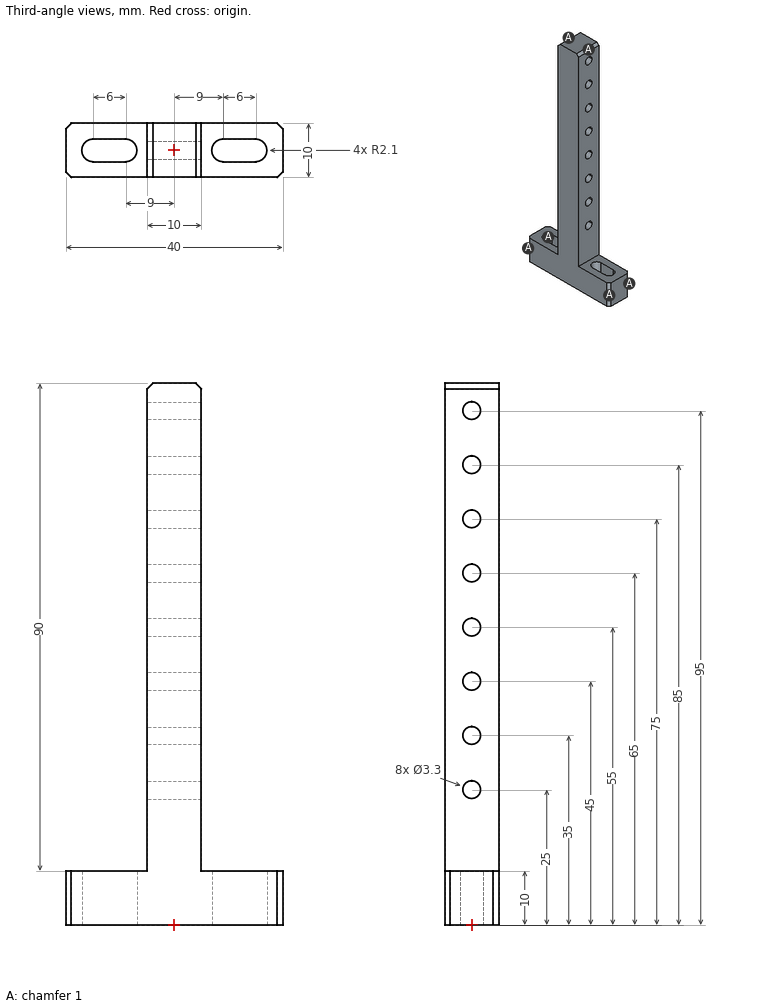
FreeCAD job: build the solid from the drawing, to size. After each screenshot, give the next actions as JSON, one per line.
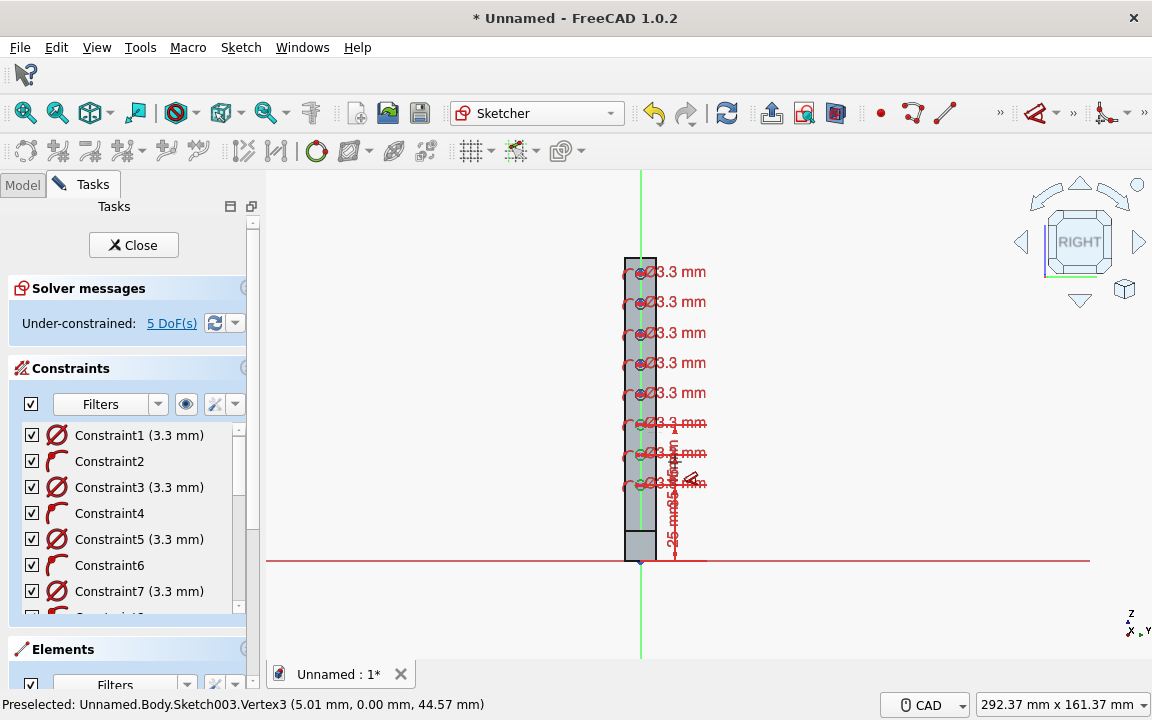
{"action": "left_click", "coordinate": [641, 395]}
{"action": "left_click", "coordinate": [675, 440]}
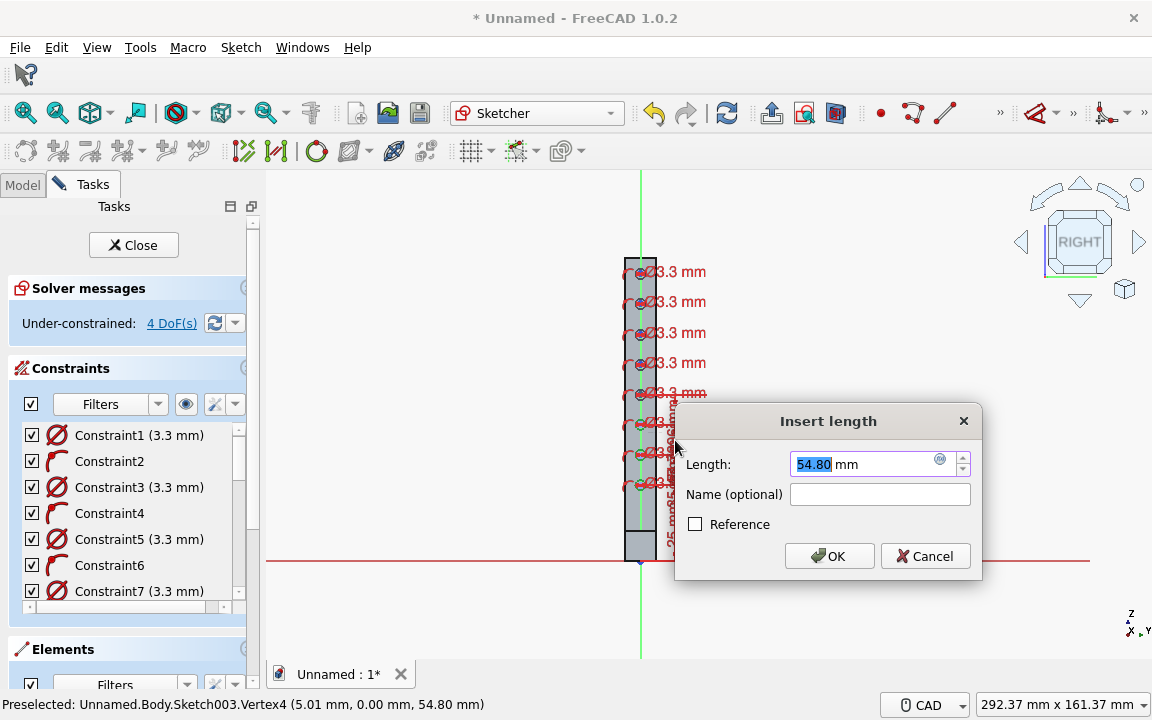
{"action": "type", "text": "55"}
{"action": "key", "text": "Return"}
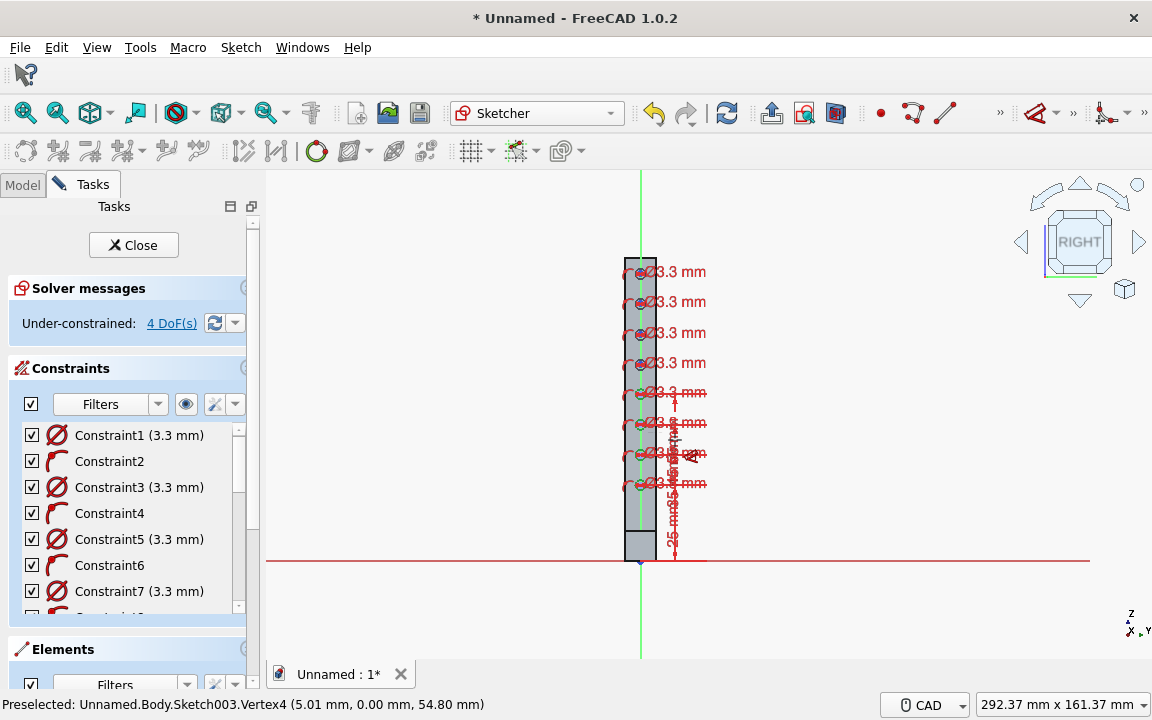
{"action": "left_click", "coordinate": [641, 365]}
{"action": "left_click", "coordinate": [675, 418]}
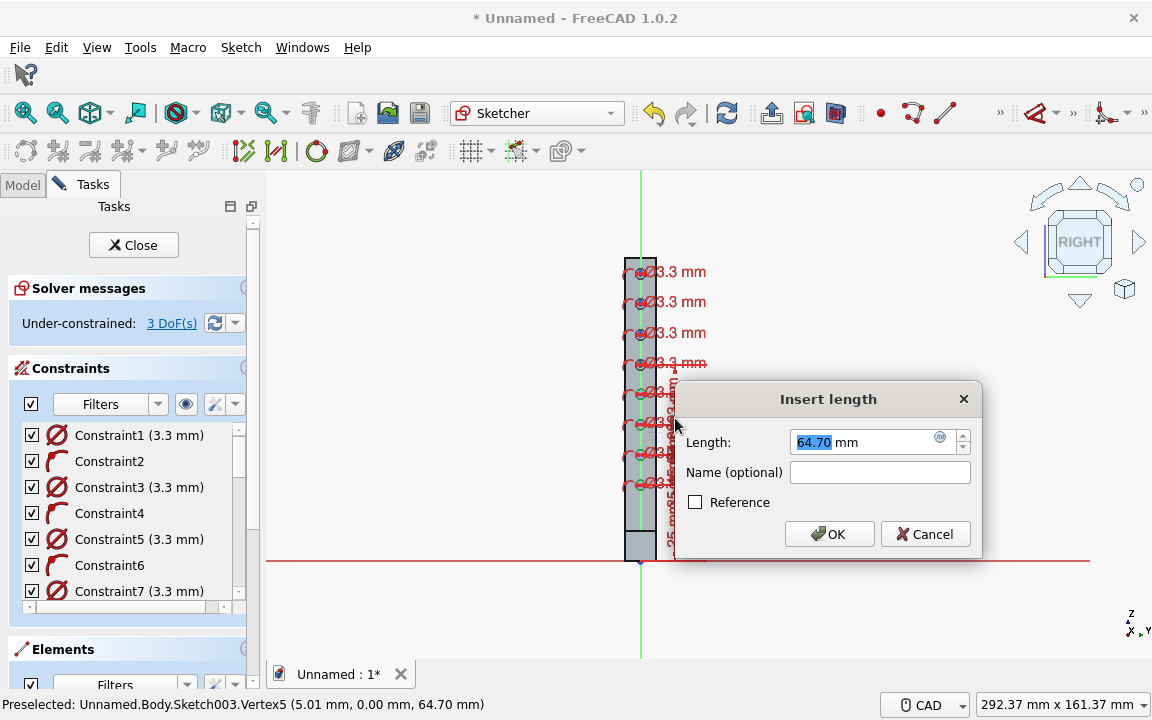
{"action": "type", "text": "65"}
{"action": "key", "text": "Return"}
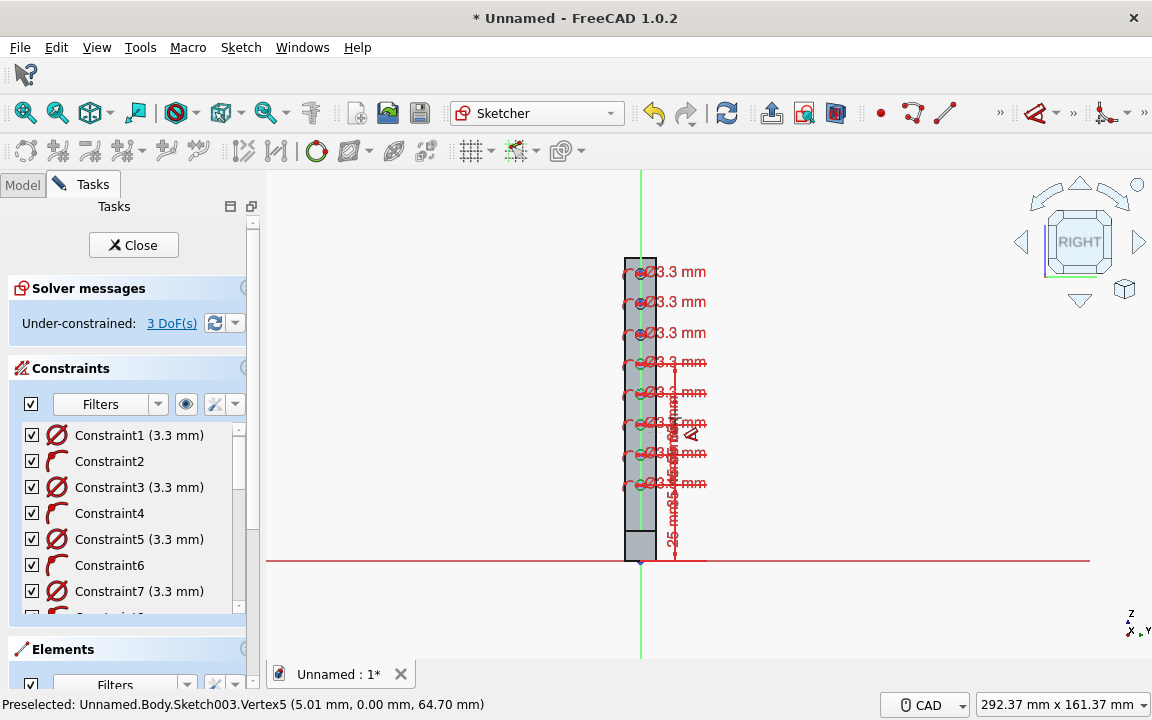
{"action": "left_click", "coordinate": [641, 335]}
{"action": "left_click", "coordinate": [675, 396]}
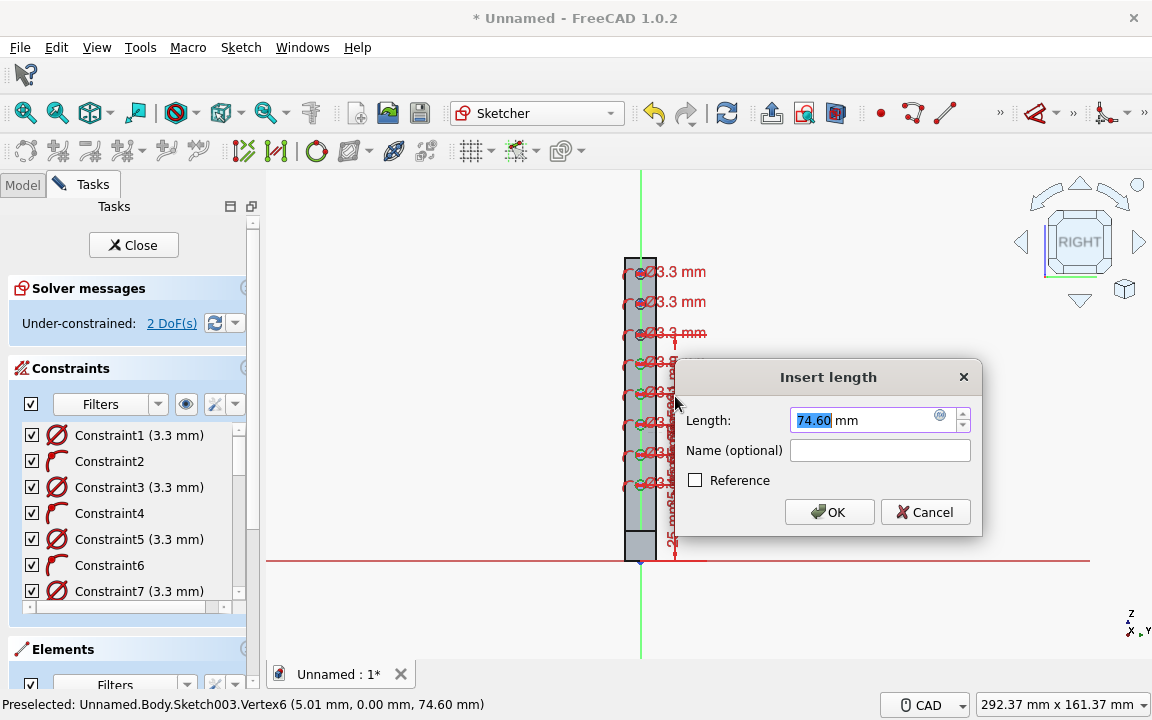
{"action": "type", "text": "75"}
{"action": "key", "text": "Return"}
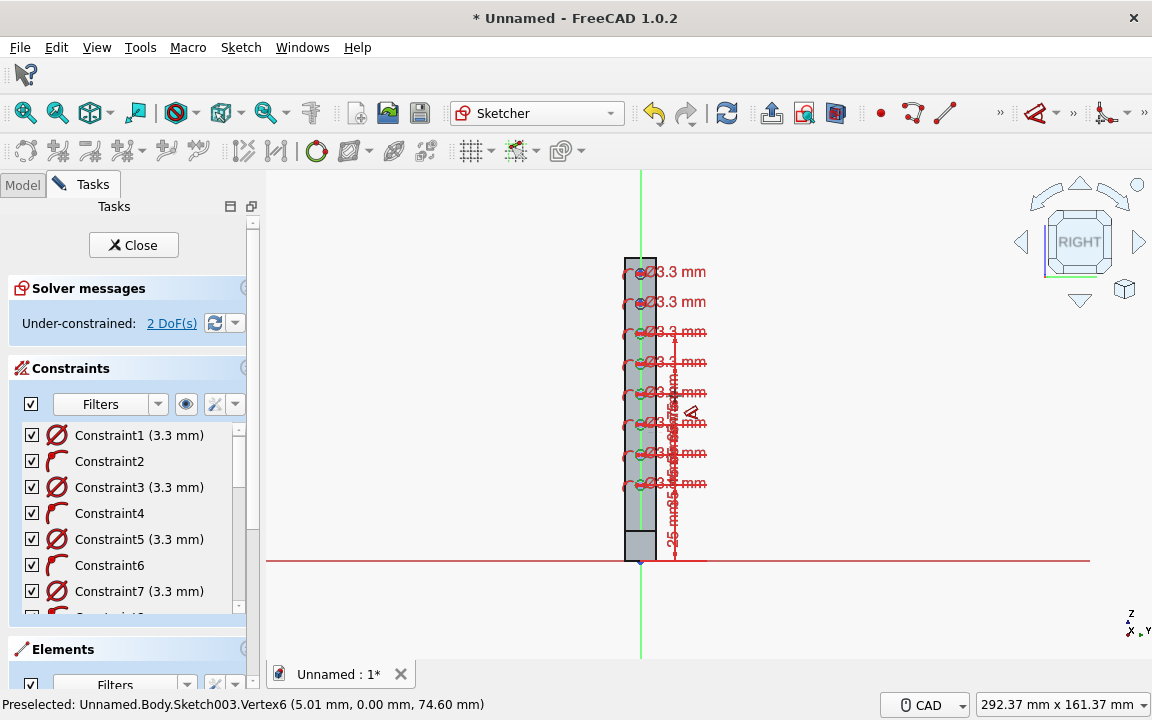
{"action": "left_click", "coordinate": [641, 304]}
{"action": "left_click", "coordinate": [675, 373]}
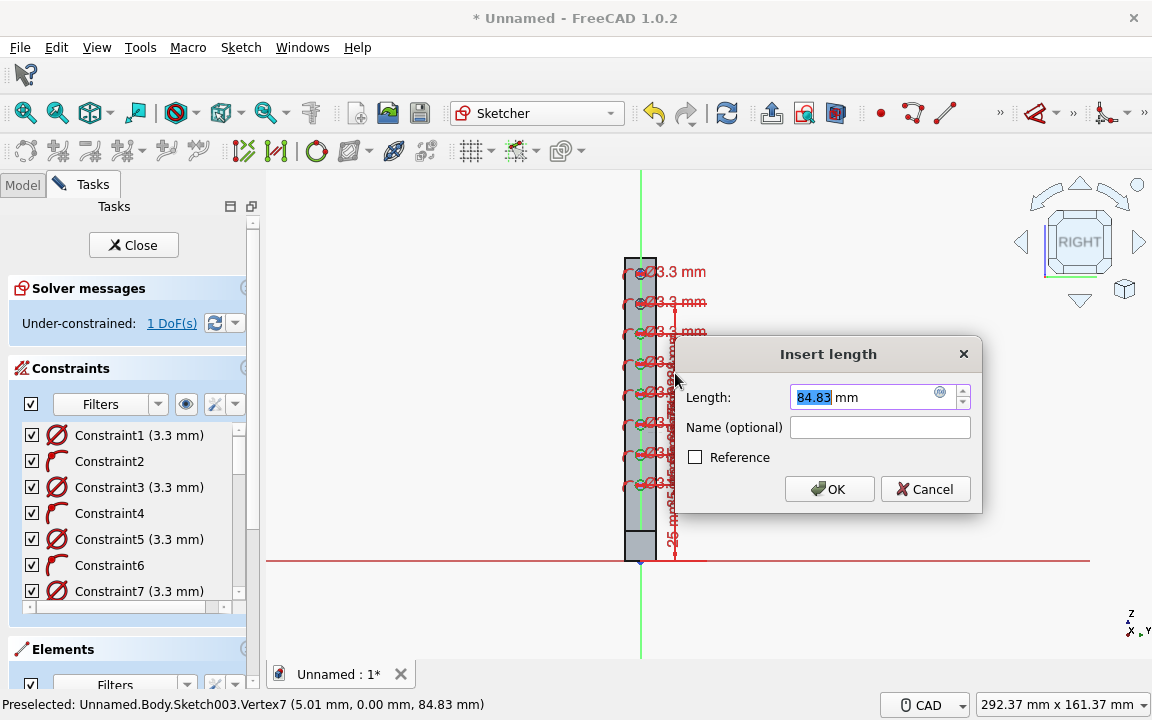
{"action": "type", "text": "85"}
{"action": "key", "text": "Return"}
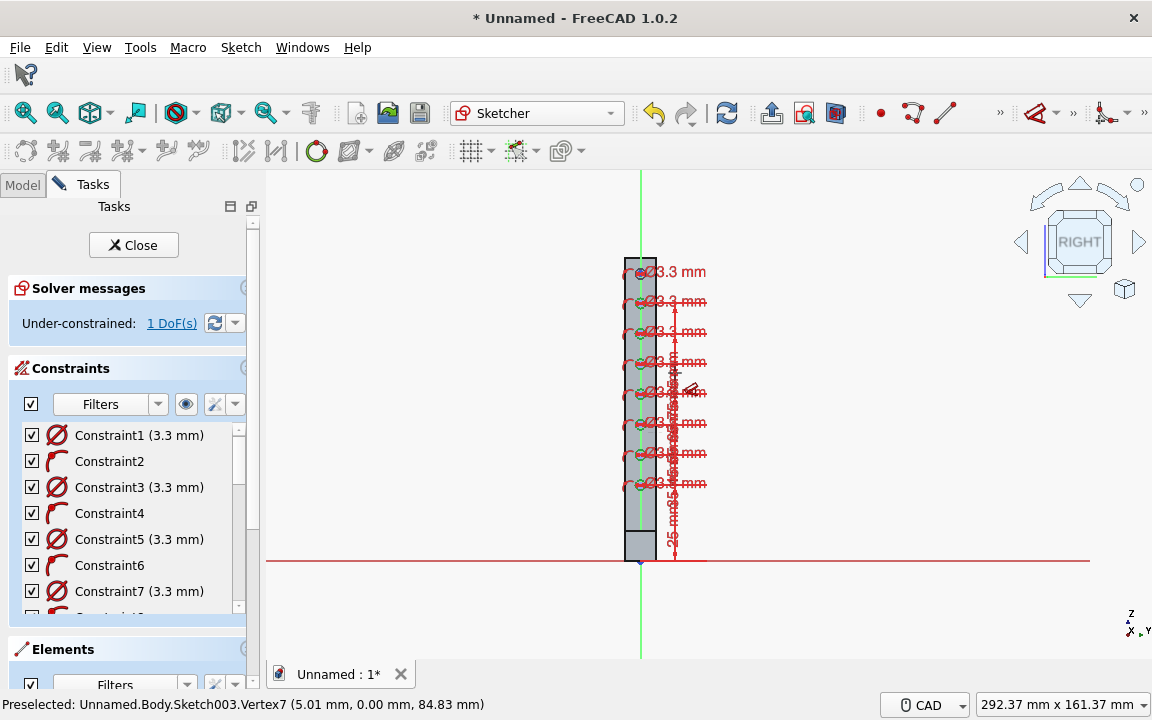
{"action": "left_click", "coordinate": [641, 274]}
{"action": "left_click", "coordinate": [675, 352]}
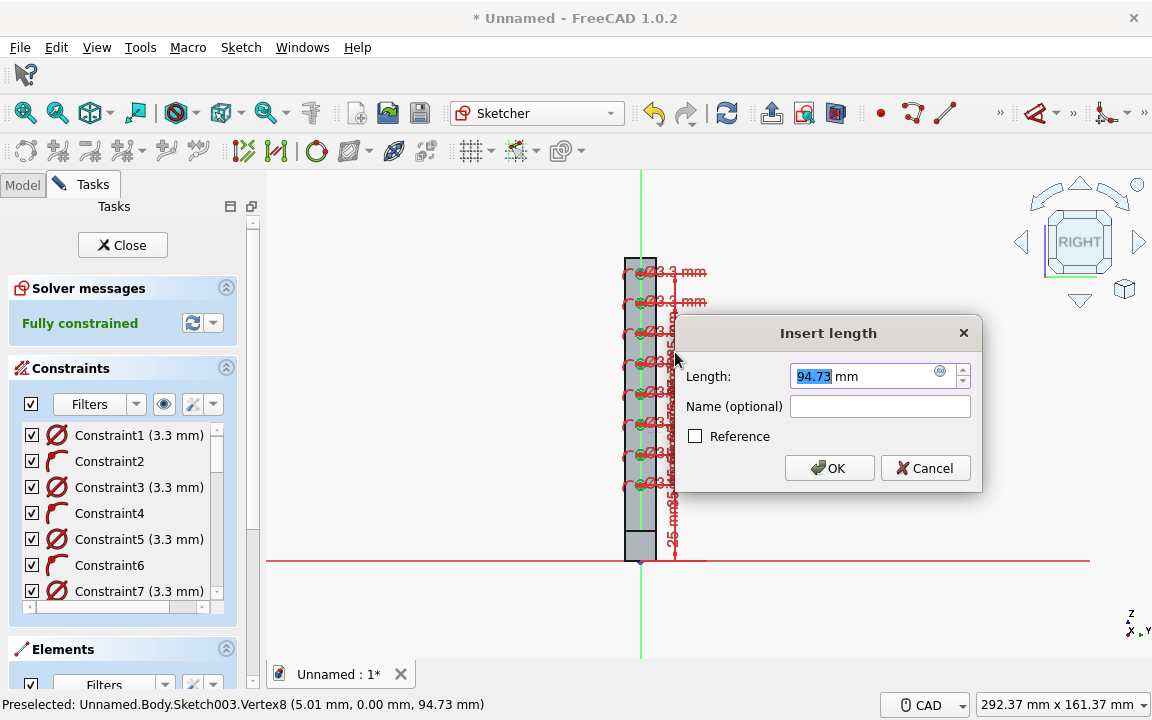
{"action": "type", "text": "95"}
{"action": "key", "text": "Return"}
{"action": "key", "text": "Escape"}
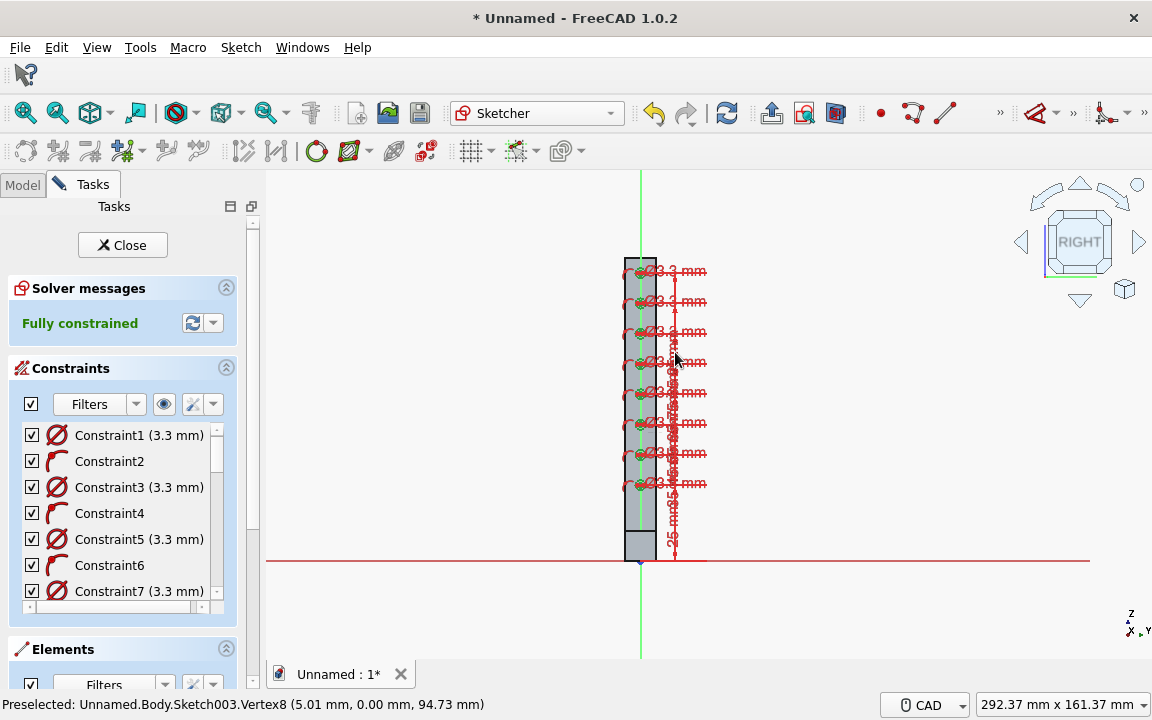
{"action": "left_click", "coordinate": [123, 245]}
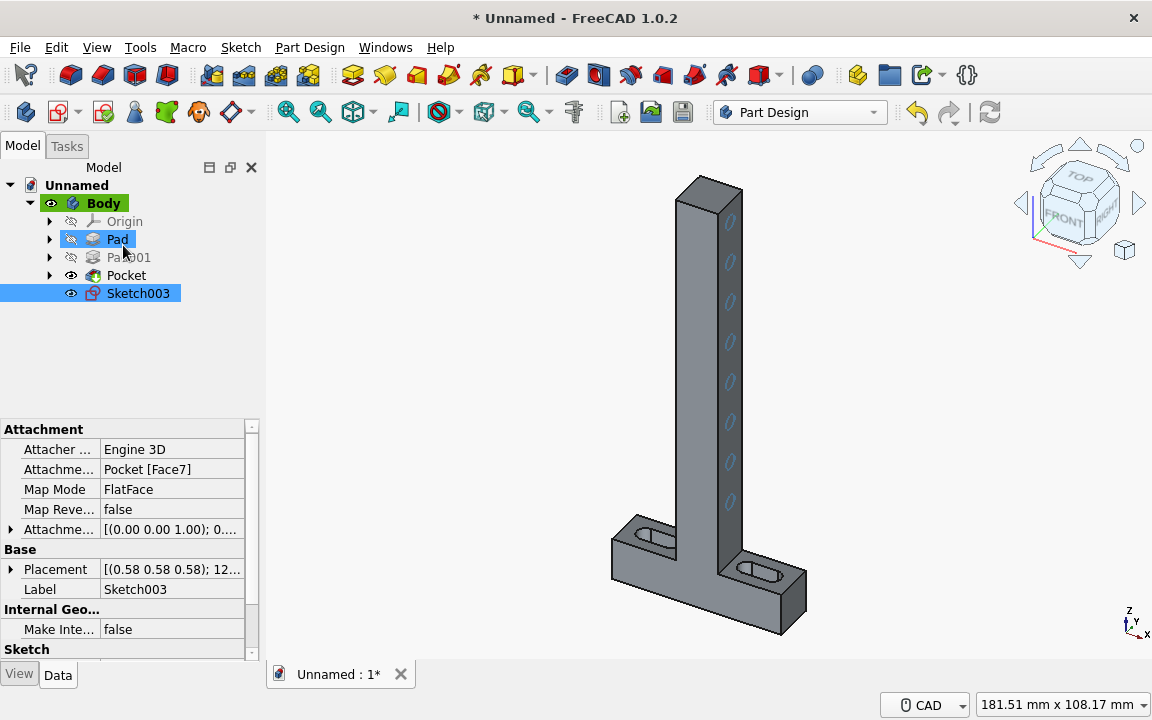
{"action": "left_click", "coordinate": [568, 76]}